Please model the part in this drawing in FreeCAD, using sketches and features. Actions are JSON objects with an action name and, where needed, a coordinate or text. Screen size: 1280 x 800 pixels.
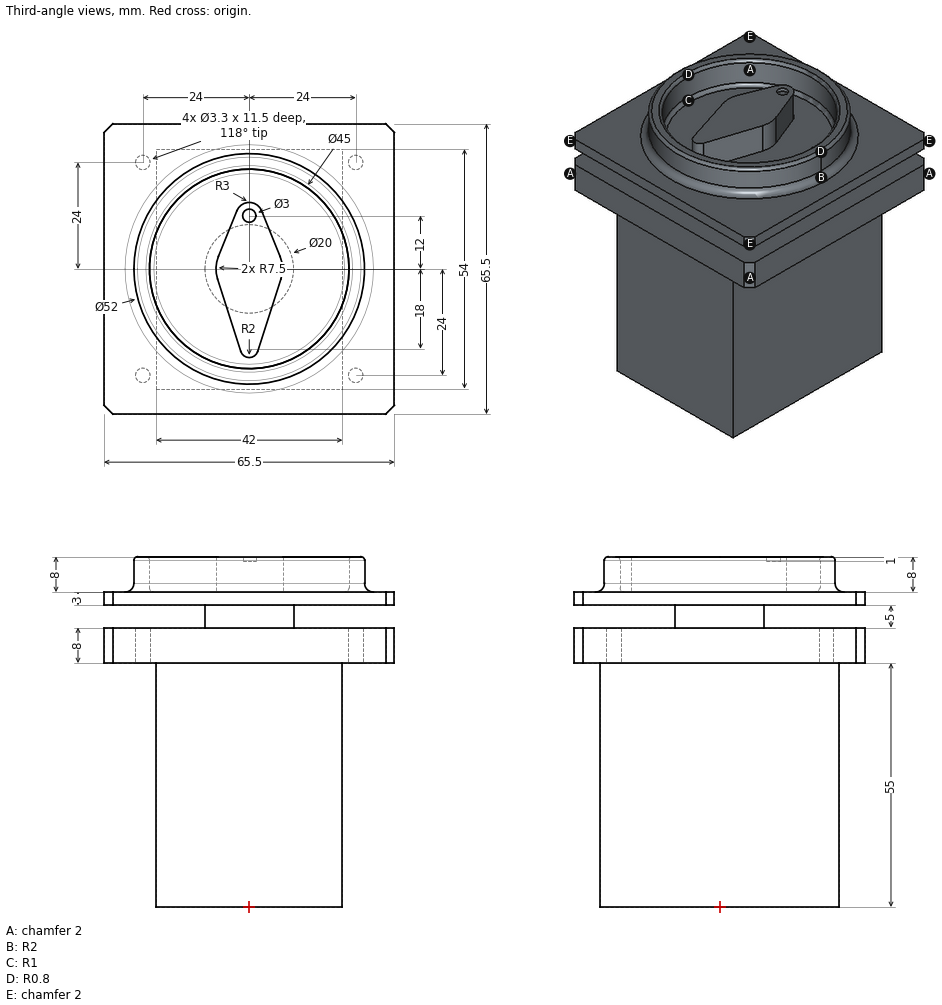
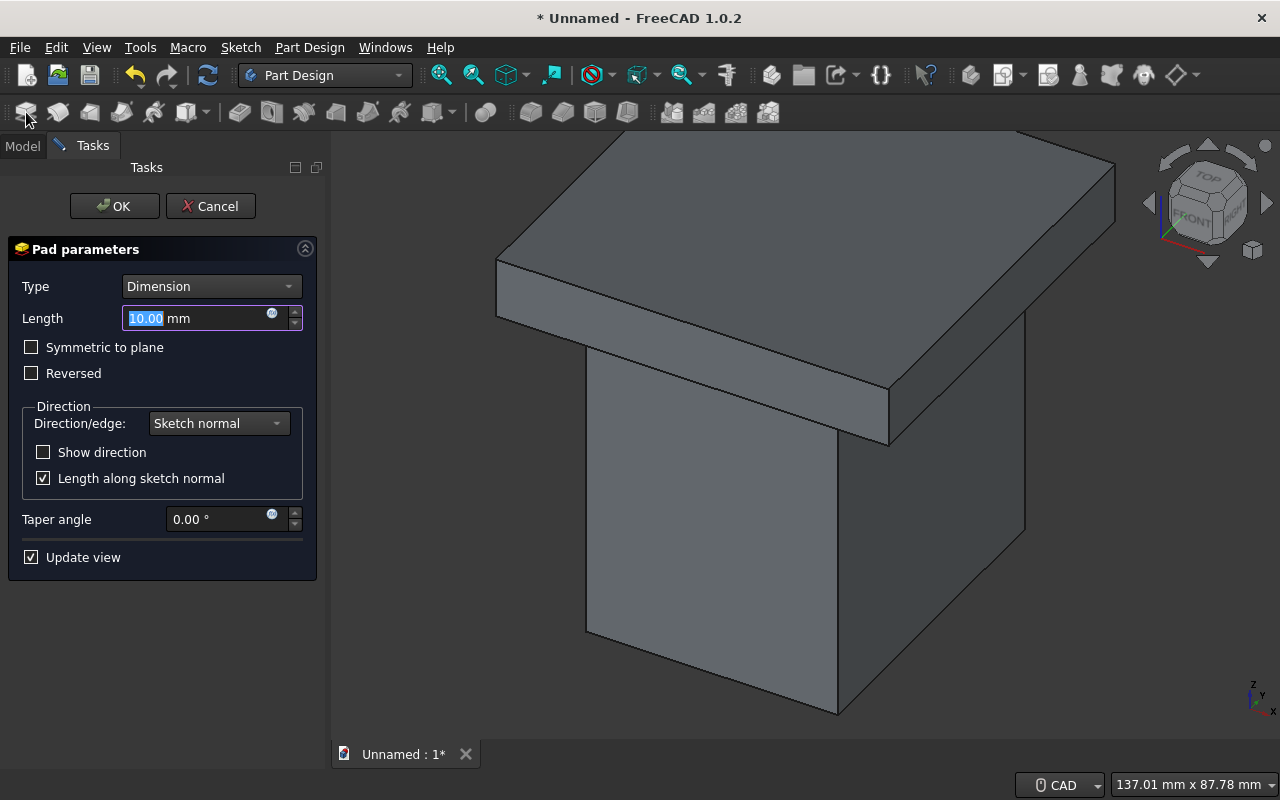
{"action": "type", "text": "8"}
{"action": "key", "text": "Tab"}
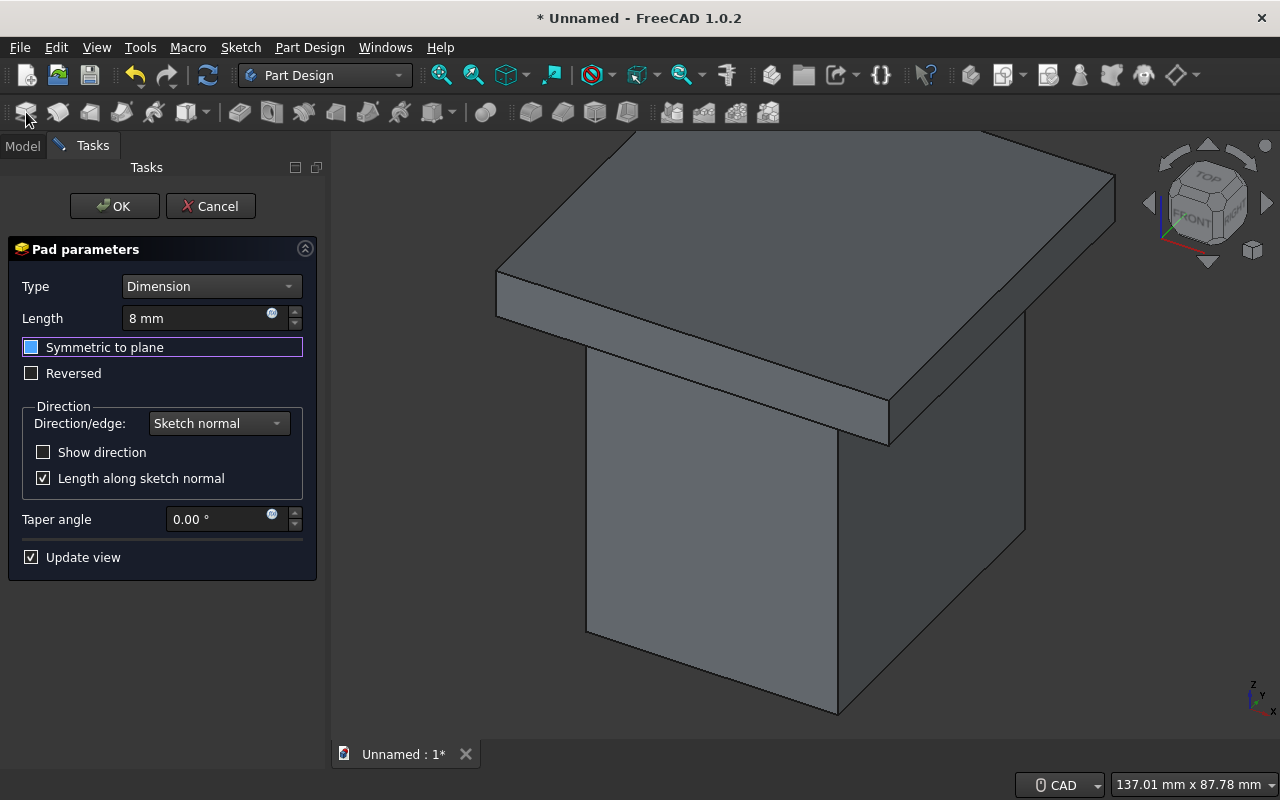
{"action": "left_click", "coordinate": [115, 206]}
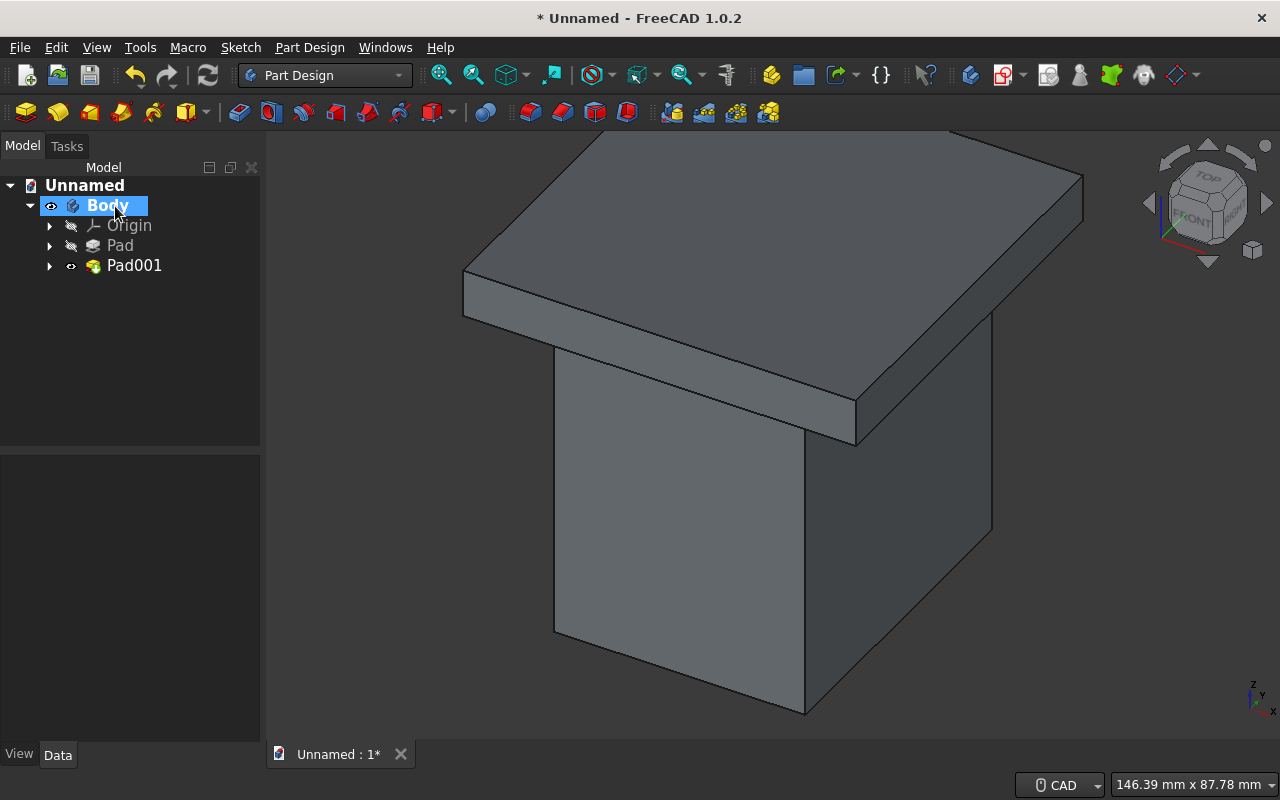
{"action": "left_click", "coordinate": [442, 76]}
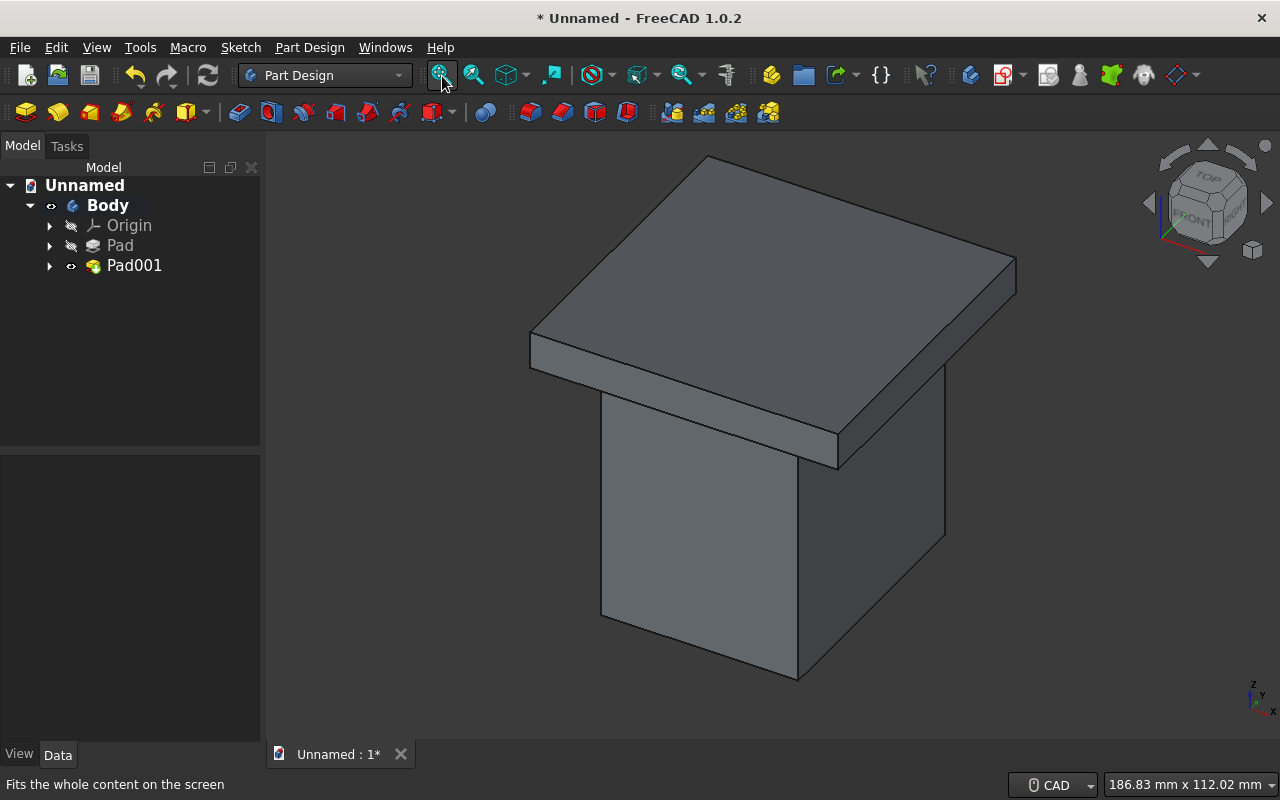
{"action": "left_click", "coordinate": [773, 294]}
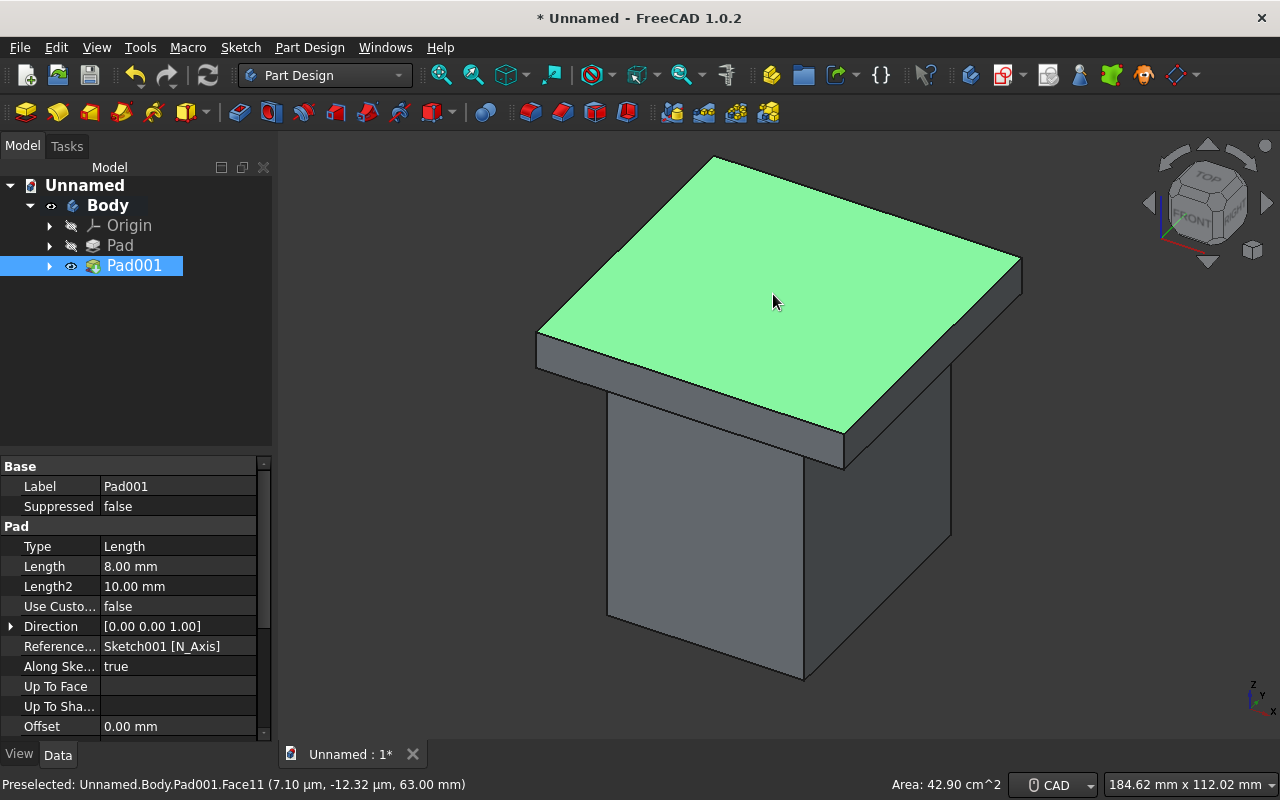
{"action": "left_click", "coordinate": [1004, 76]}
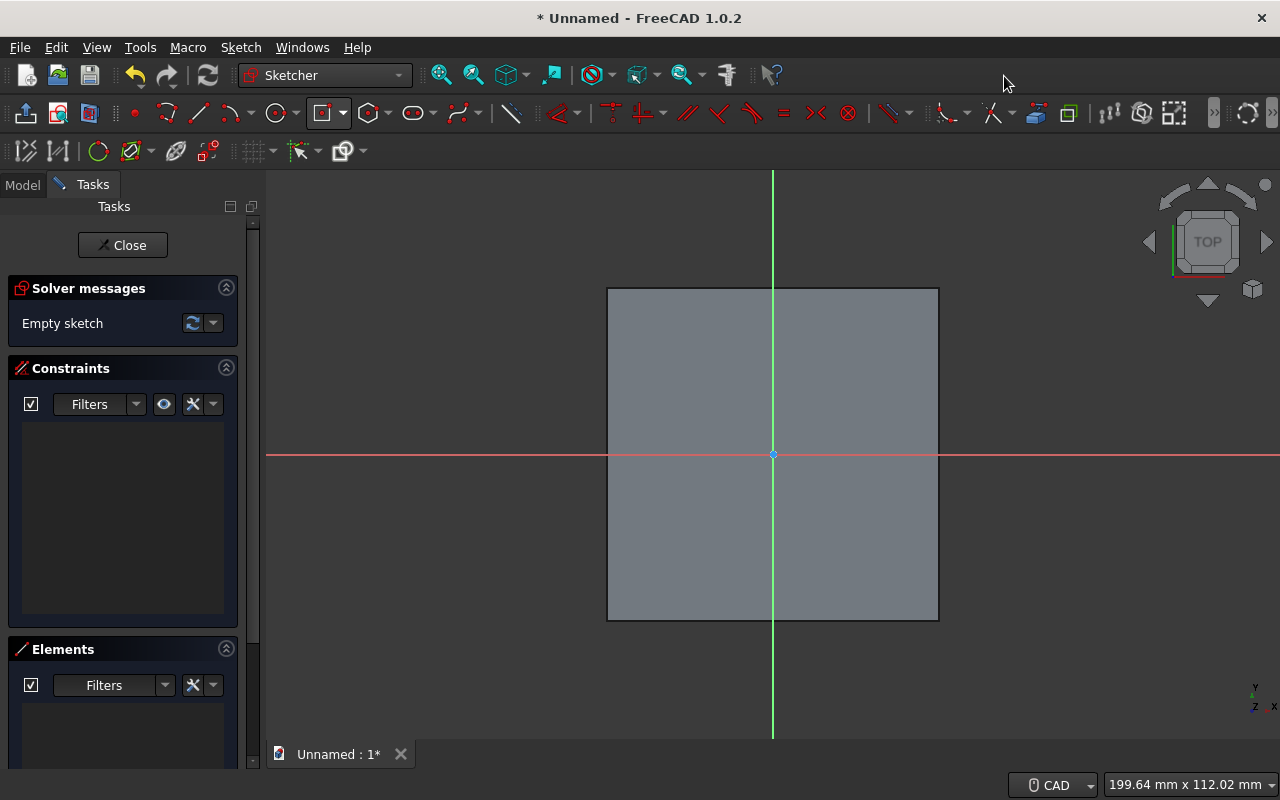
{"action": "scroll", "coordinate": [803, 455], "scroll_direction": "up", "scroll_amount": 6}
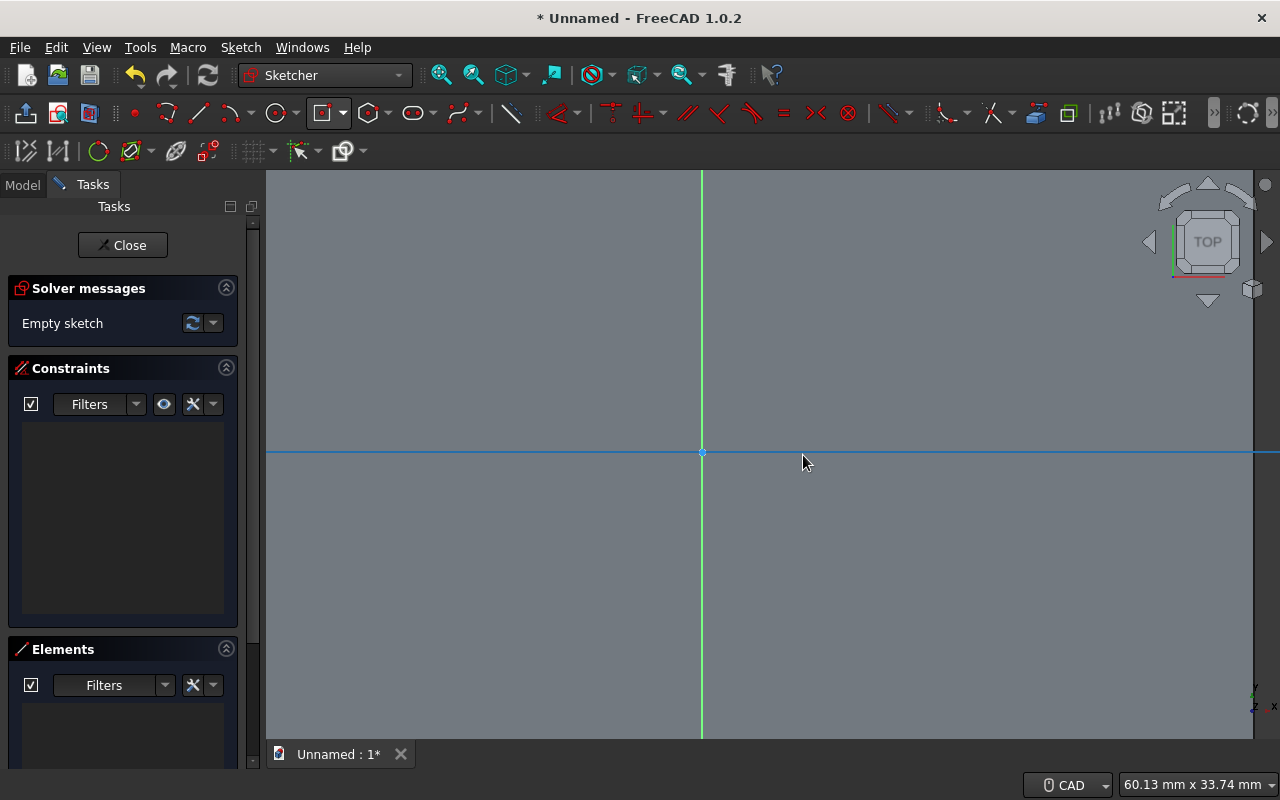
{"action": "left_click", "coordinate": [276, 114]}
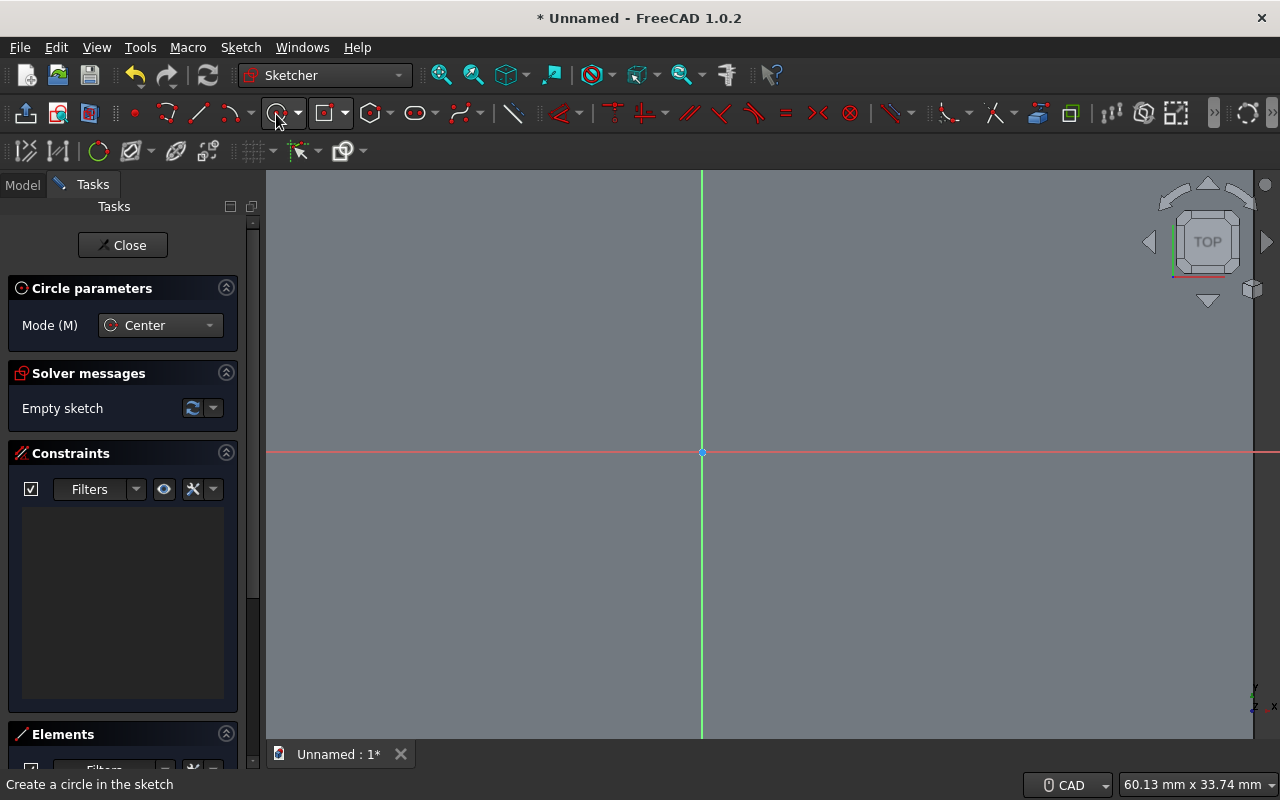
{"action": "left_click", "coordinate": [702, 452]}
{"action": "mouse_move", "coordinate": [821, 333]}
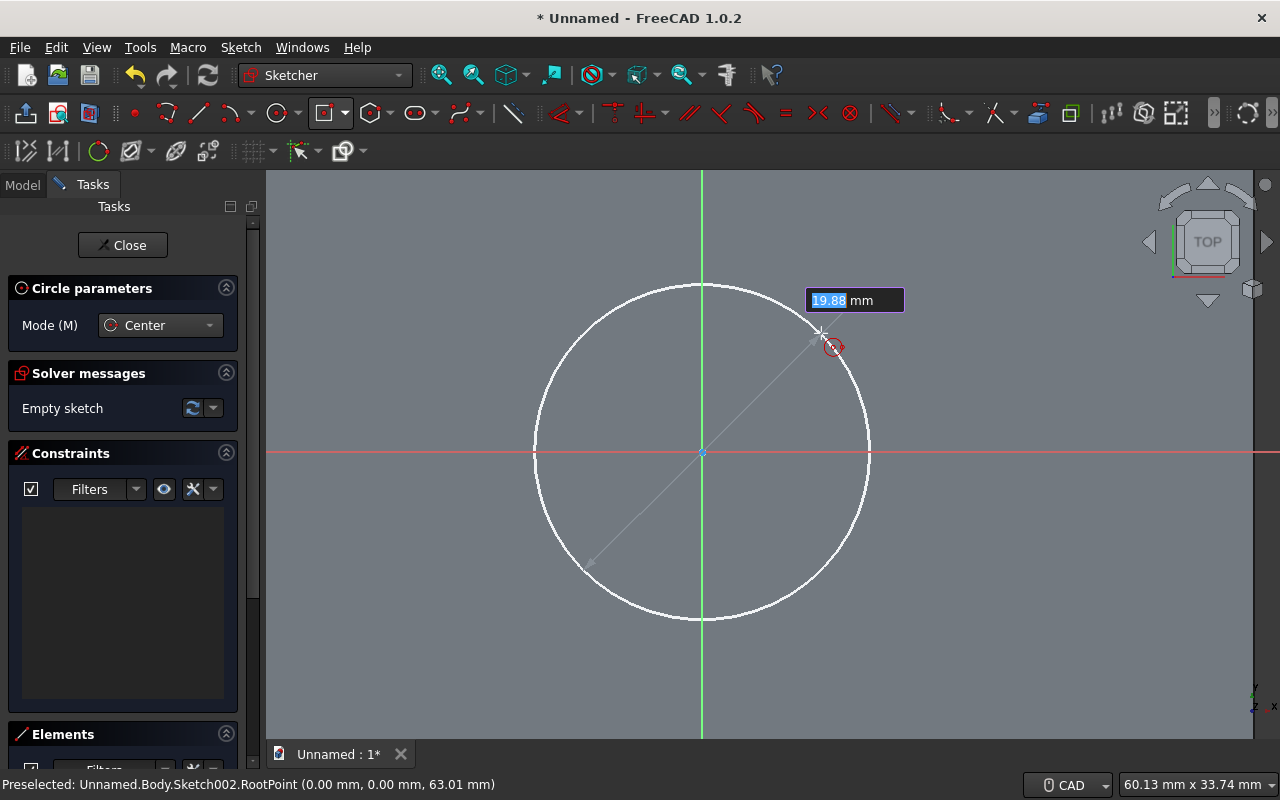
{"action": "type", "text": "20"}
{"action": "key", "text": "Return"}
{"action": "key", "text": "Escape"}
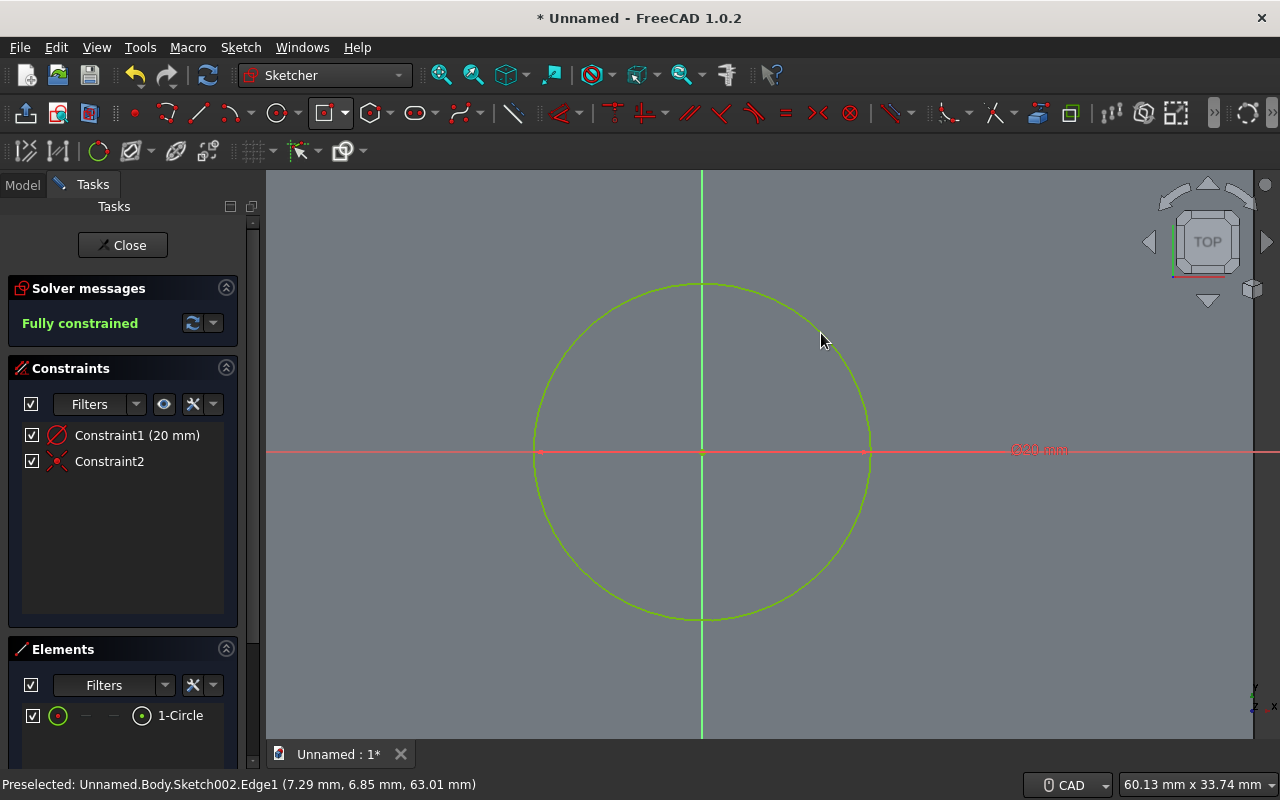
{"action": "left_click", "coordinate": [123, 245]}